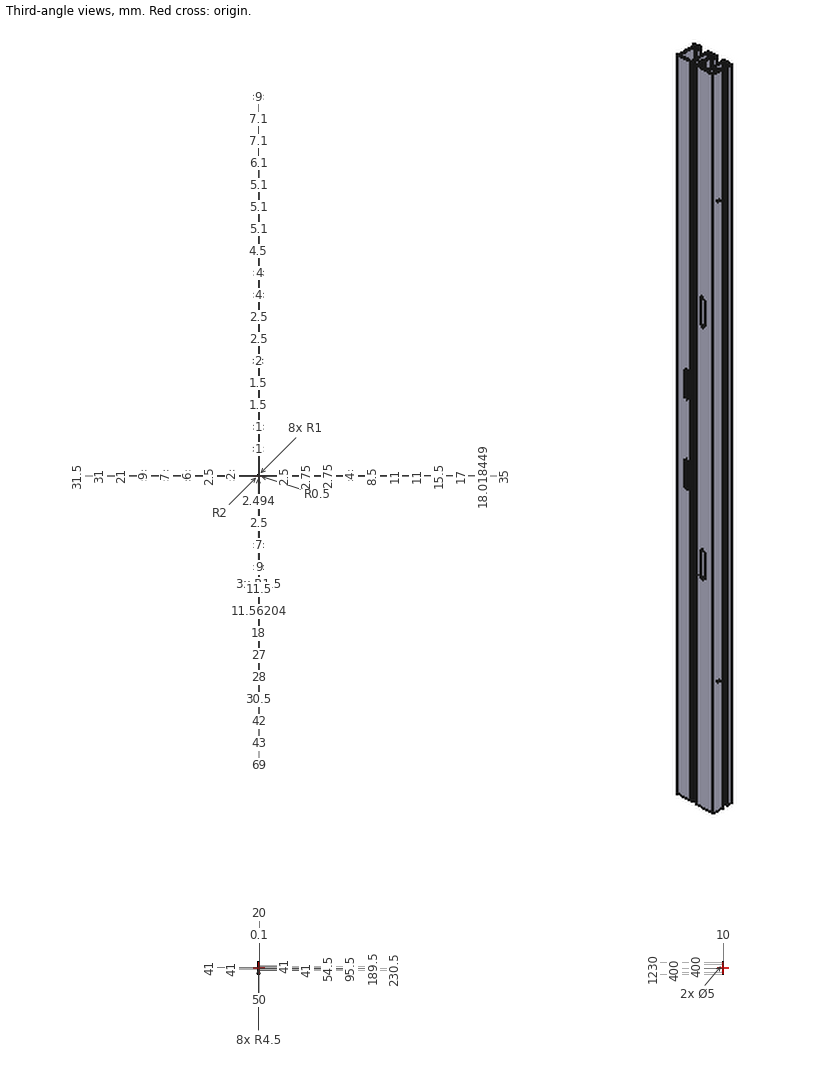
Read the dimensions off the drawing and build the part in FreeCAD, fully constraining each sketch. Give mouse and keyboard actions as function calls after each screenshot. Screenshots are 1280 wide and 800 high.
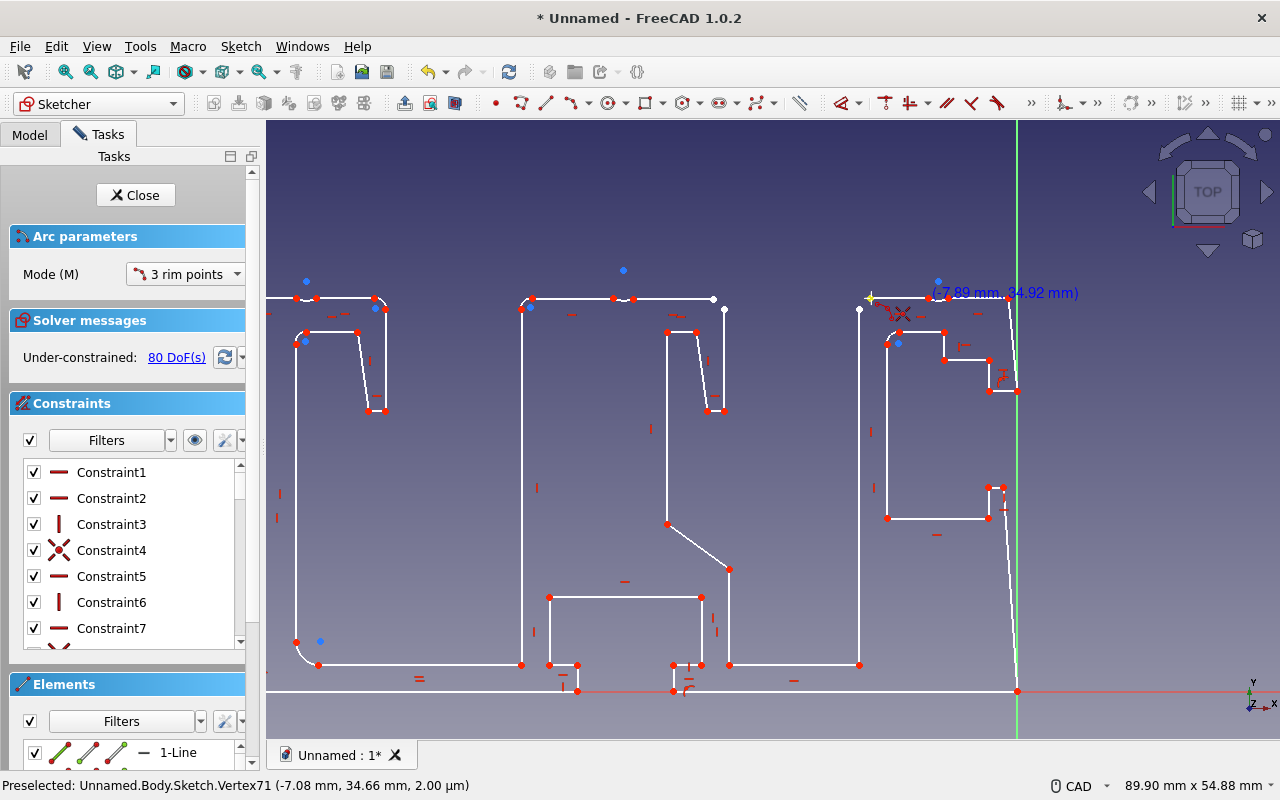
click(870, 298)
click(859, 309)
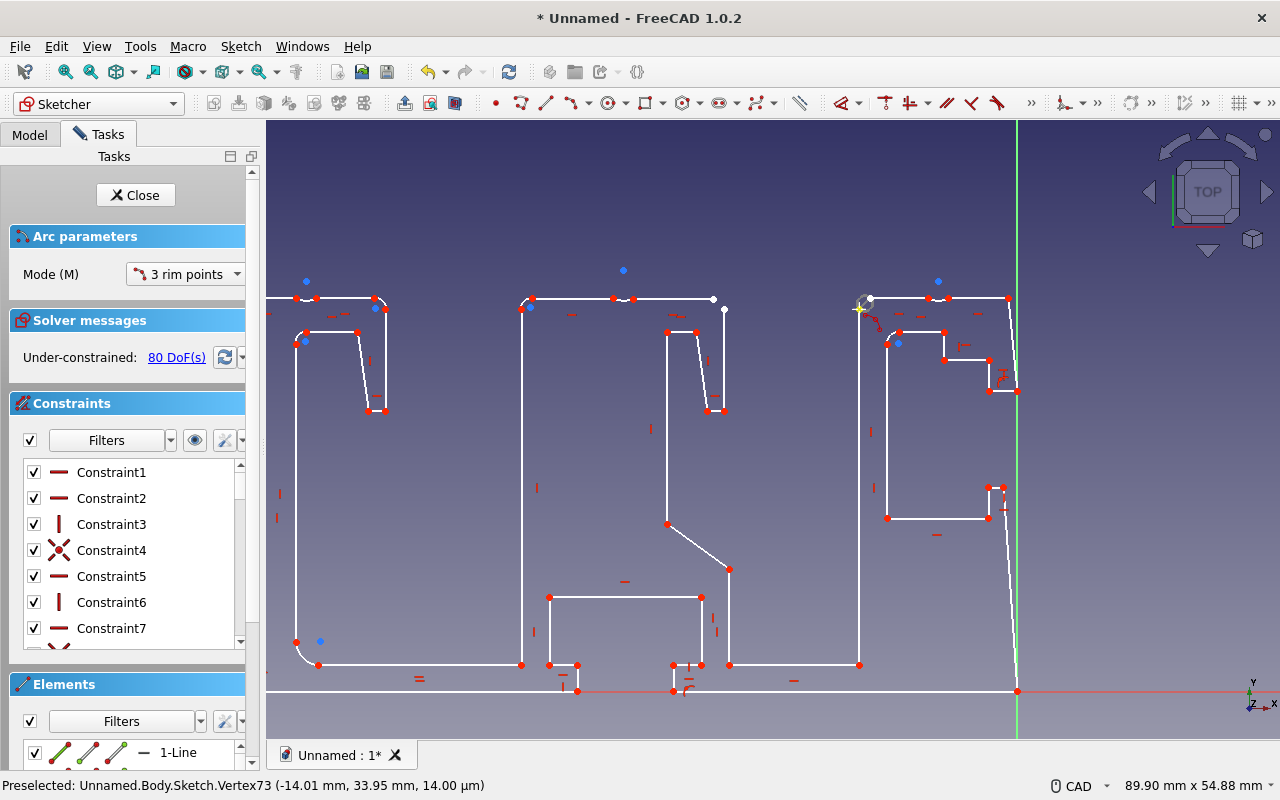
scroll(863, 300, up, 8)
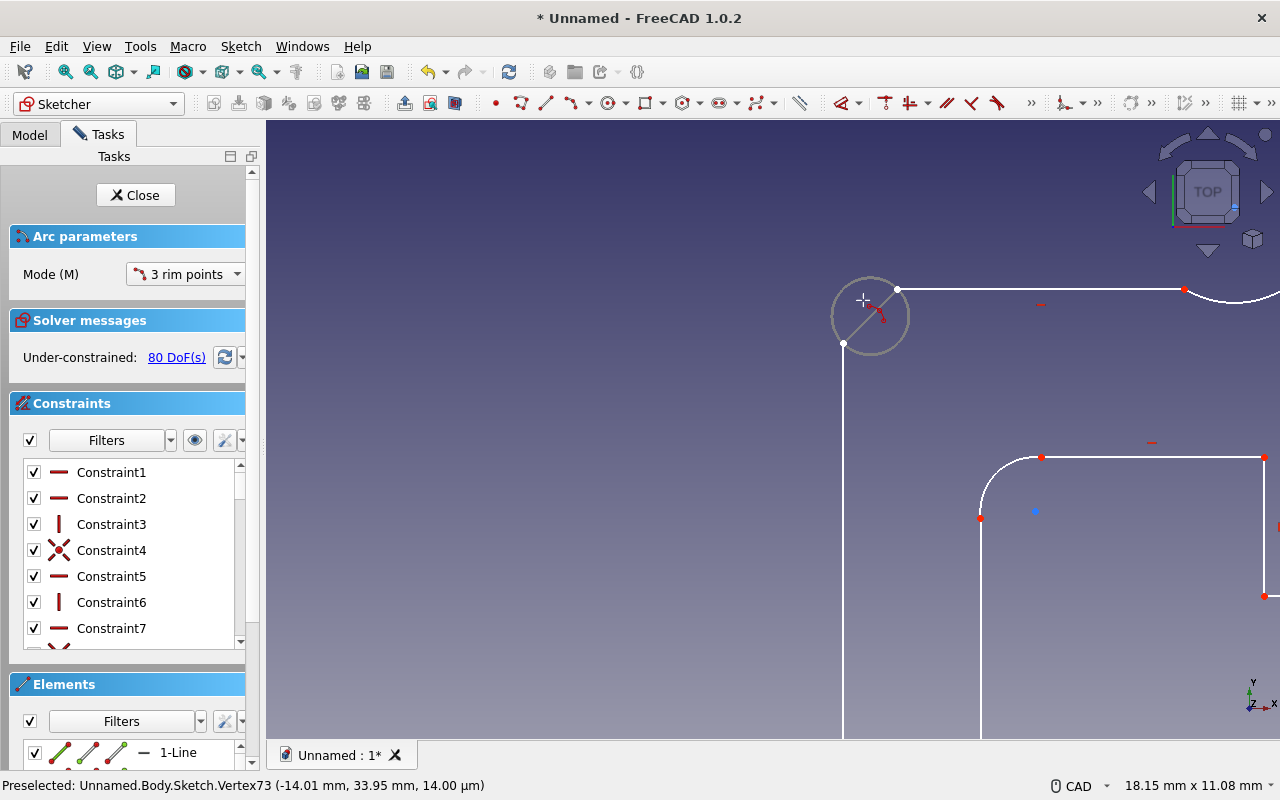
click(860, 301)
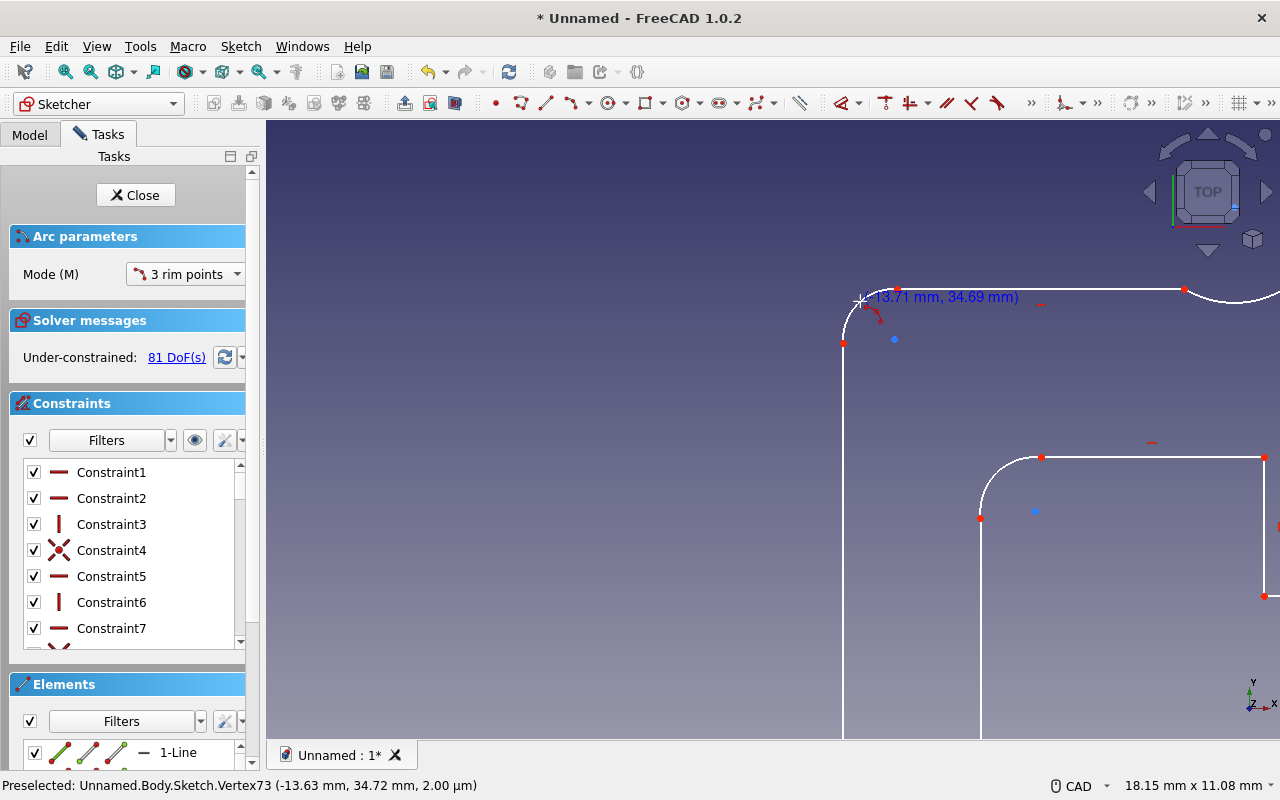
scroll(866, 299, down, 10)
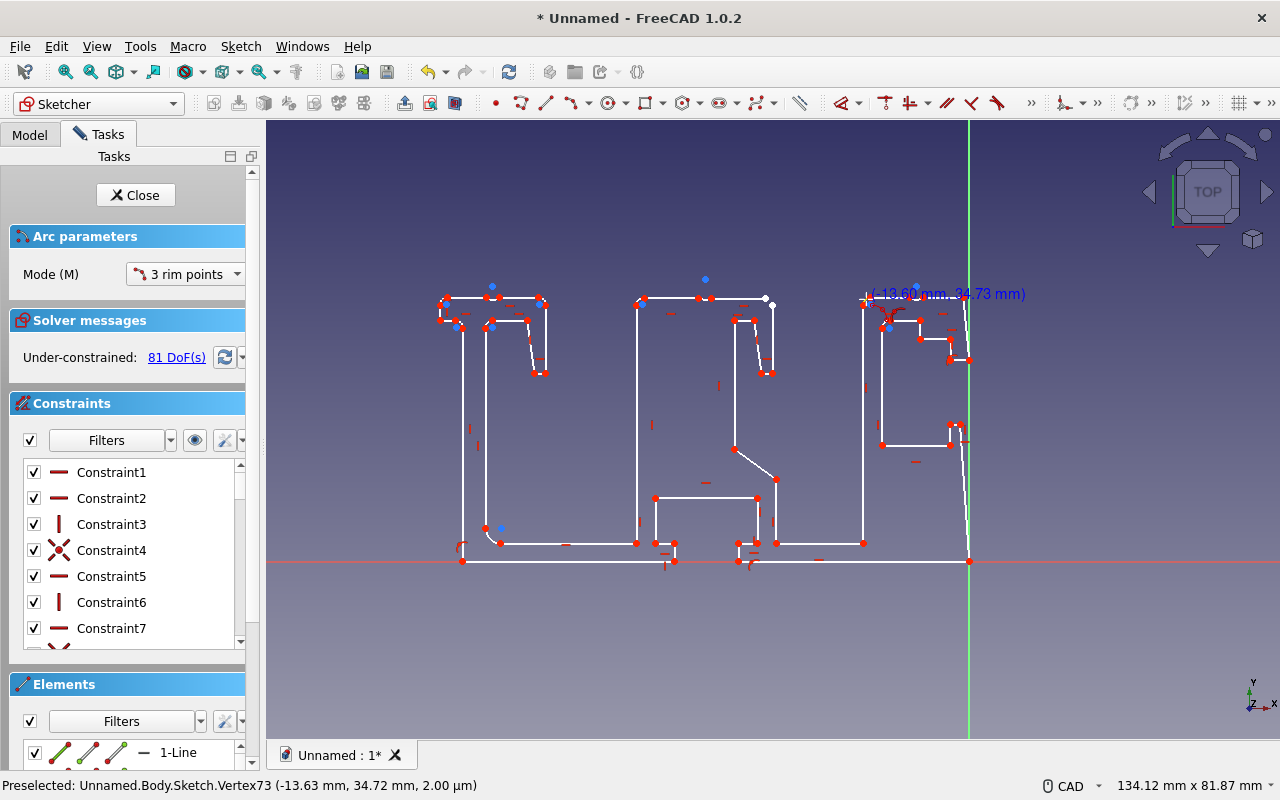
scroll(773, 305, up, 2)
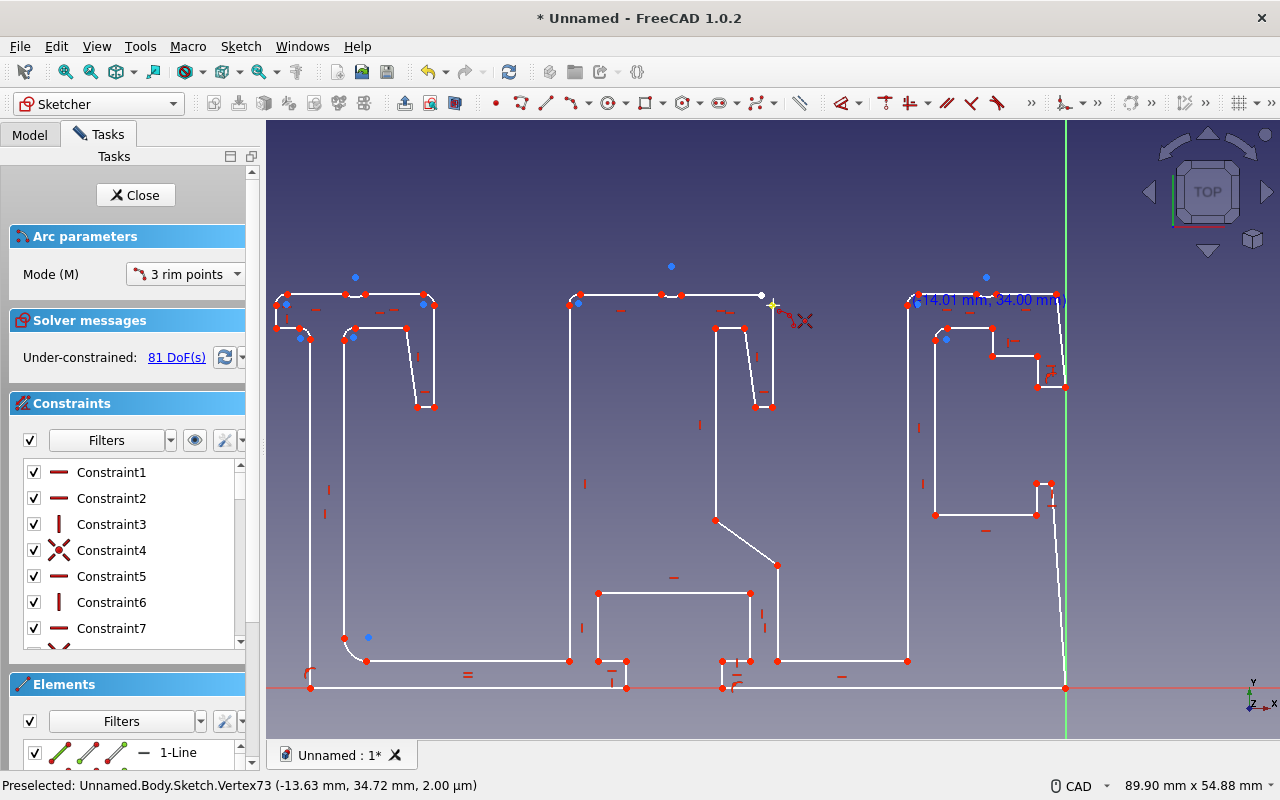
click(773, 305)
click(761, 295)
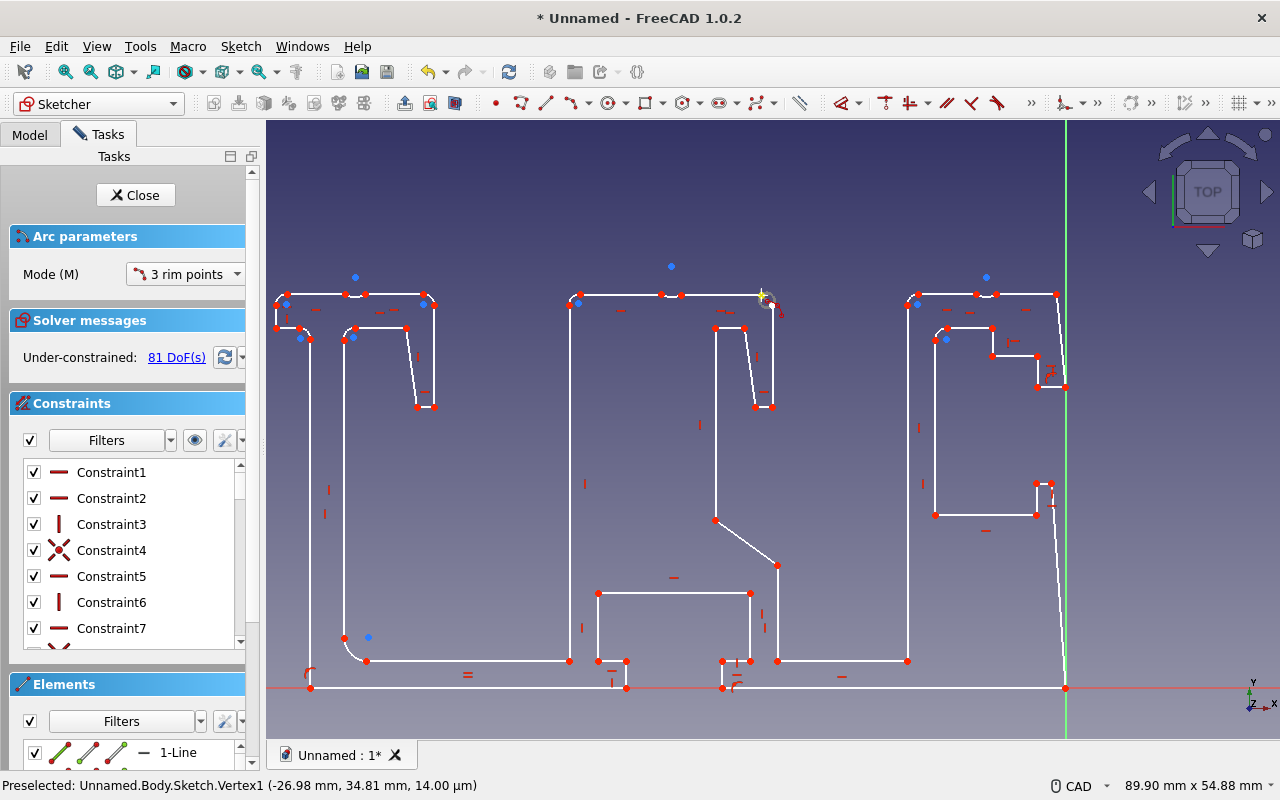
scroll(769, 297, up, 8)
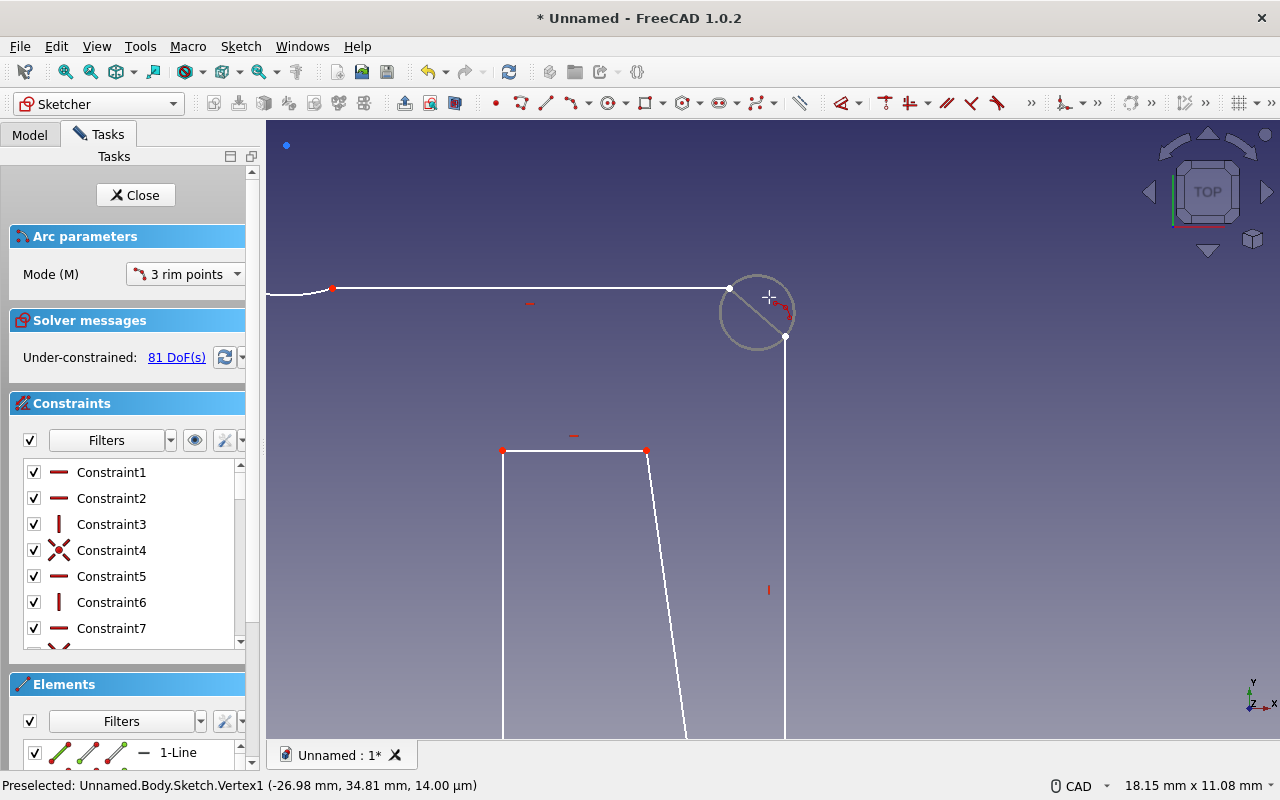
click(768, 294)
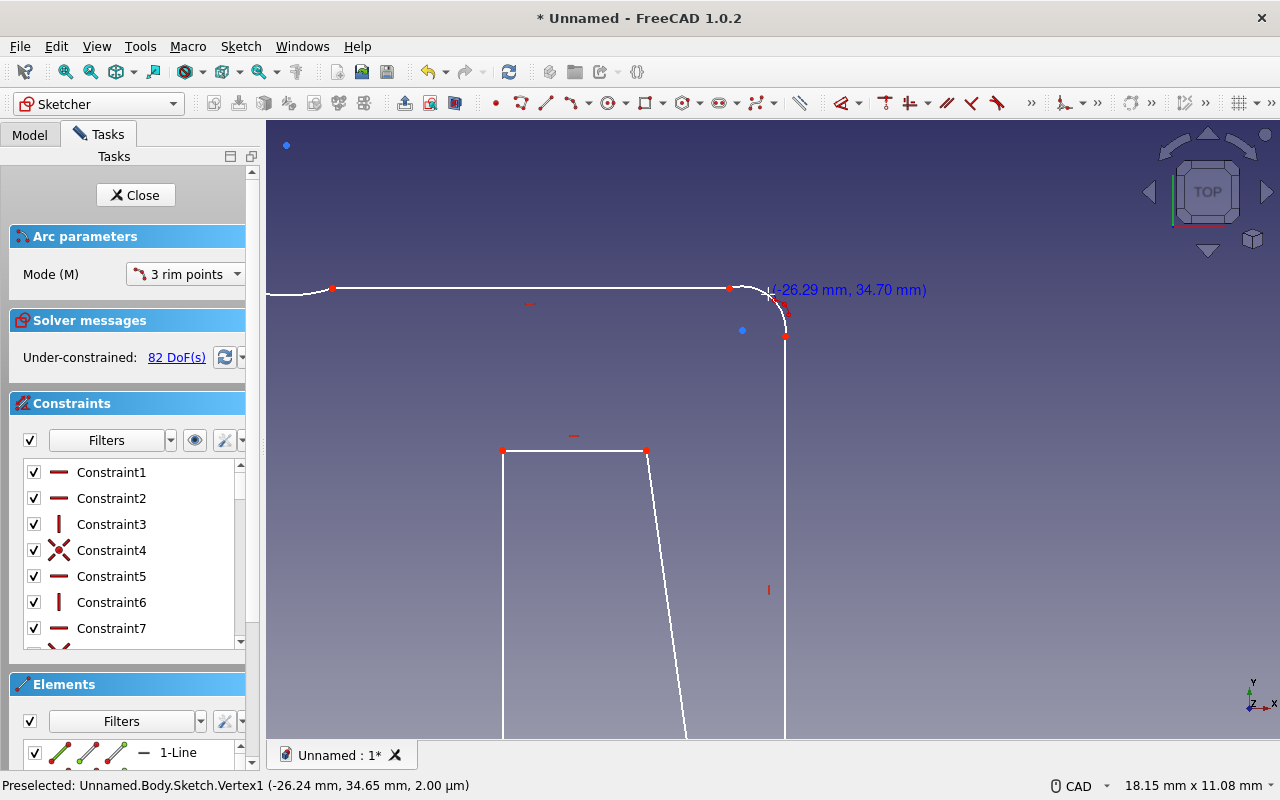
click(644, 104)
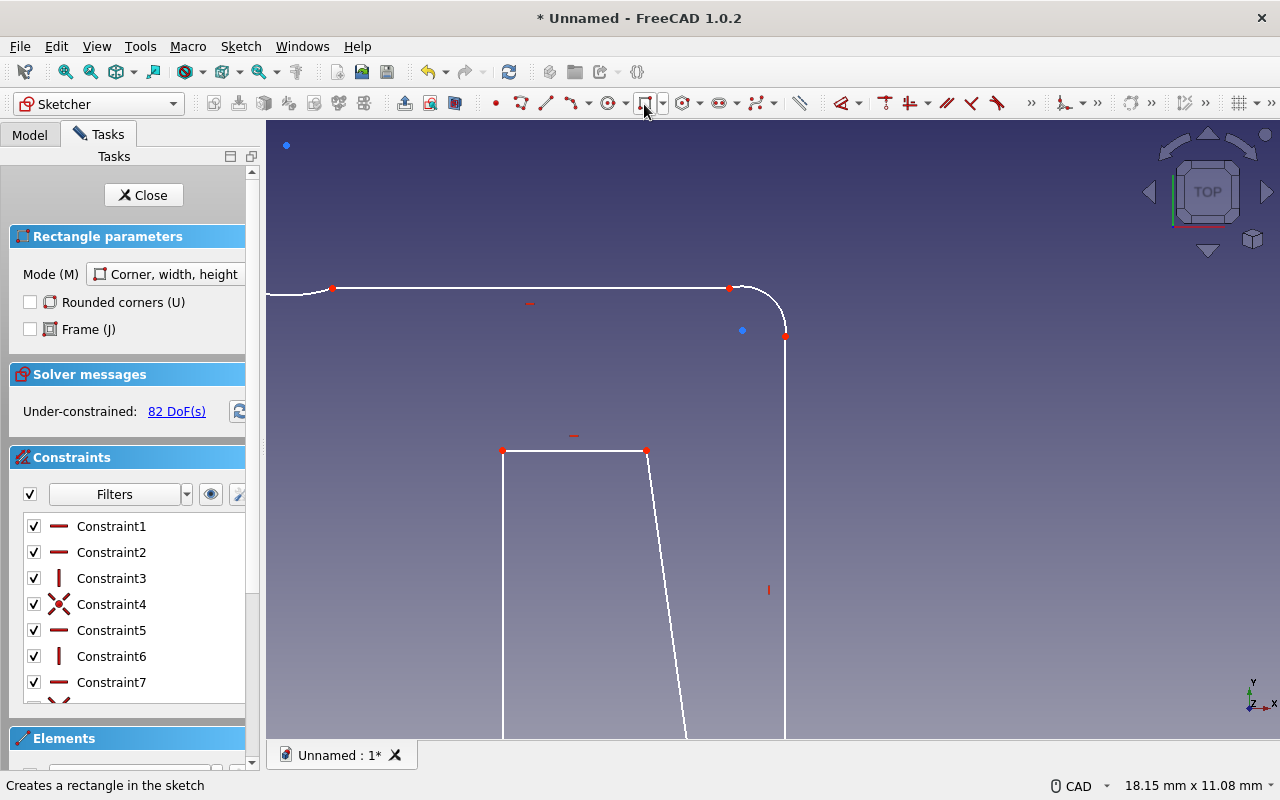
scroll(771, 300, down, 10)